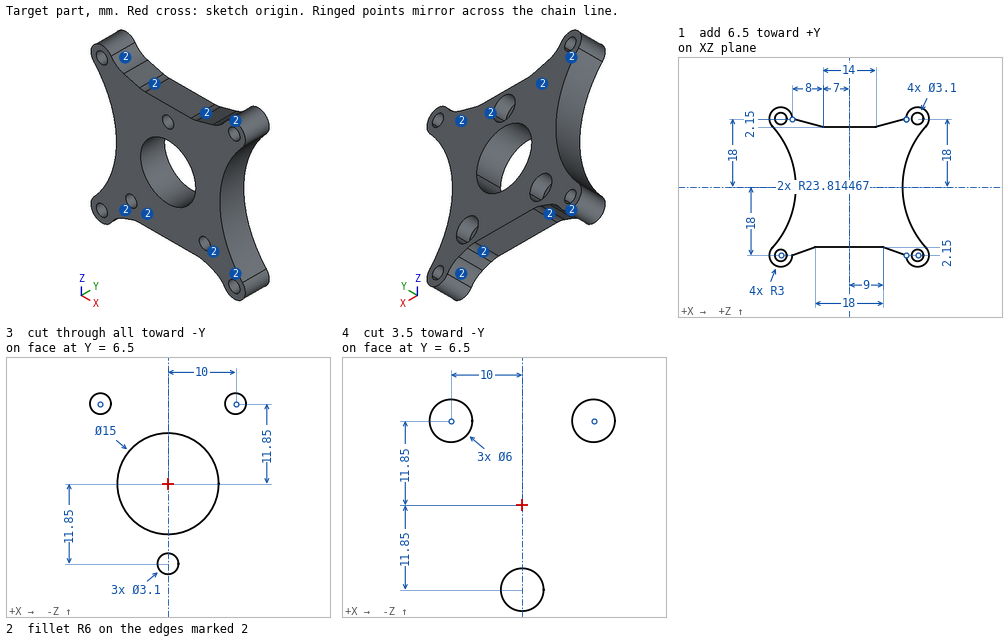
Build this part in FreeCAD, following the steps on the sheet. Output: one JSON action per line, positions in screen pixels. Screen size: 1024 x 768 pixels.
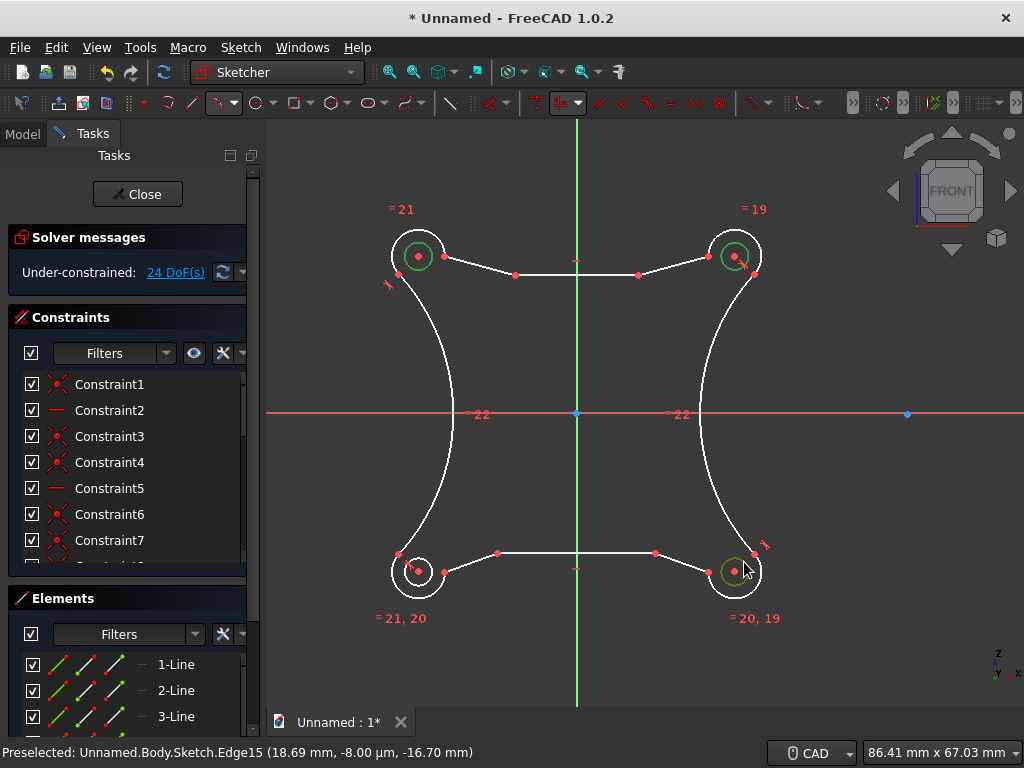
{"action": "left_click", "coordinate": [428, 562]}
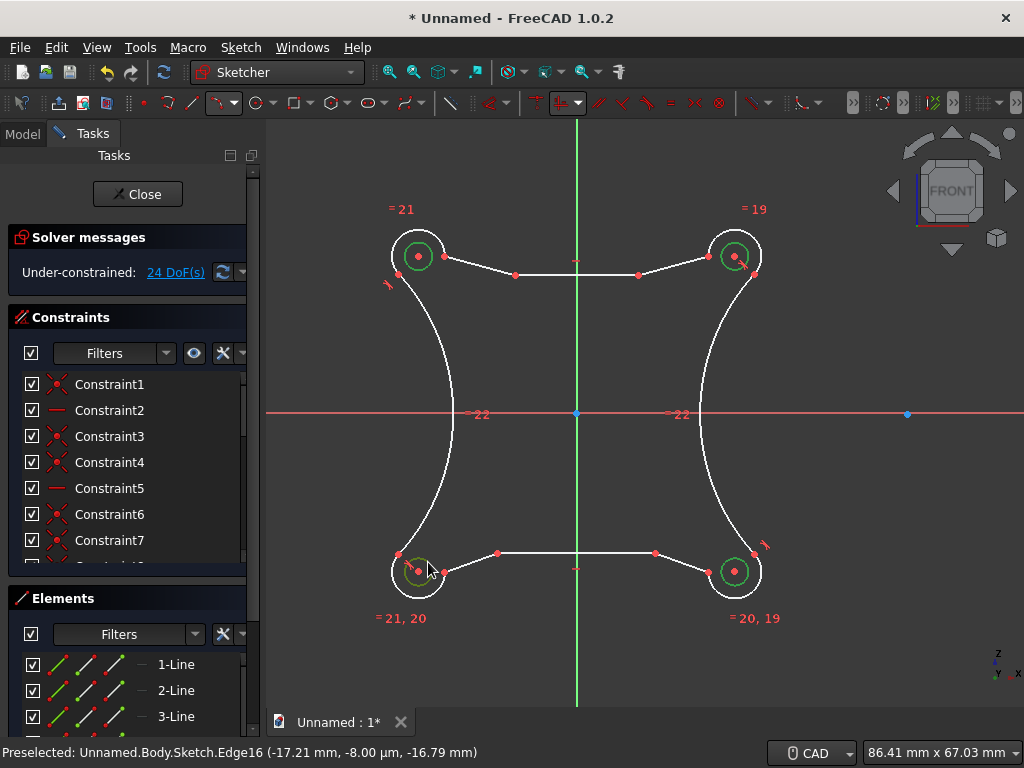
{"action": "left_click", "coordinate": [672, 104]}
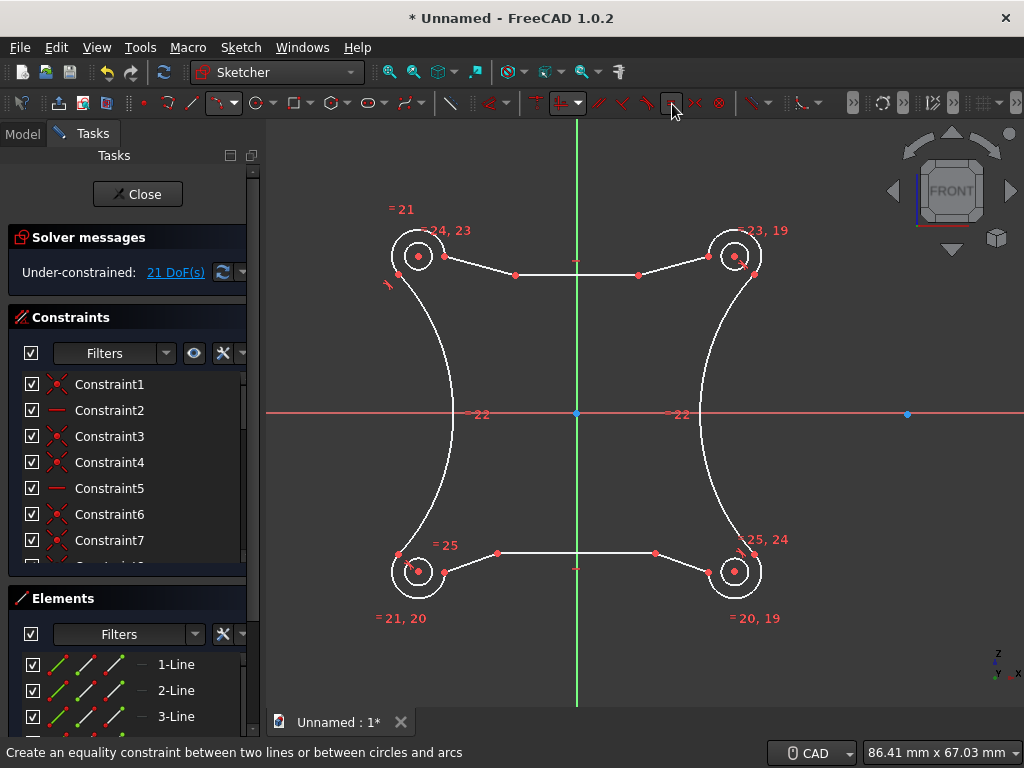
{"action": "scroll", "coordinate": [294, 412], "scroll_direction": "down", "scroll_amount": 1}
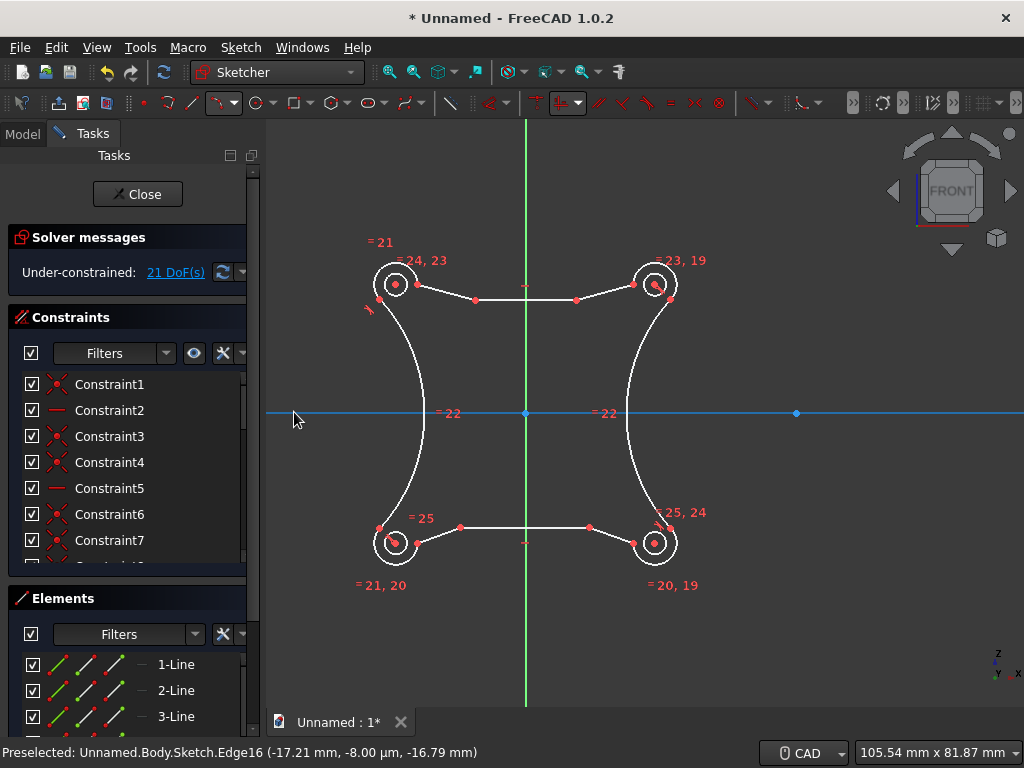
{"action": "left_click", "coordinate": [796, 414]}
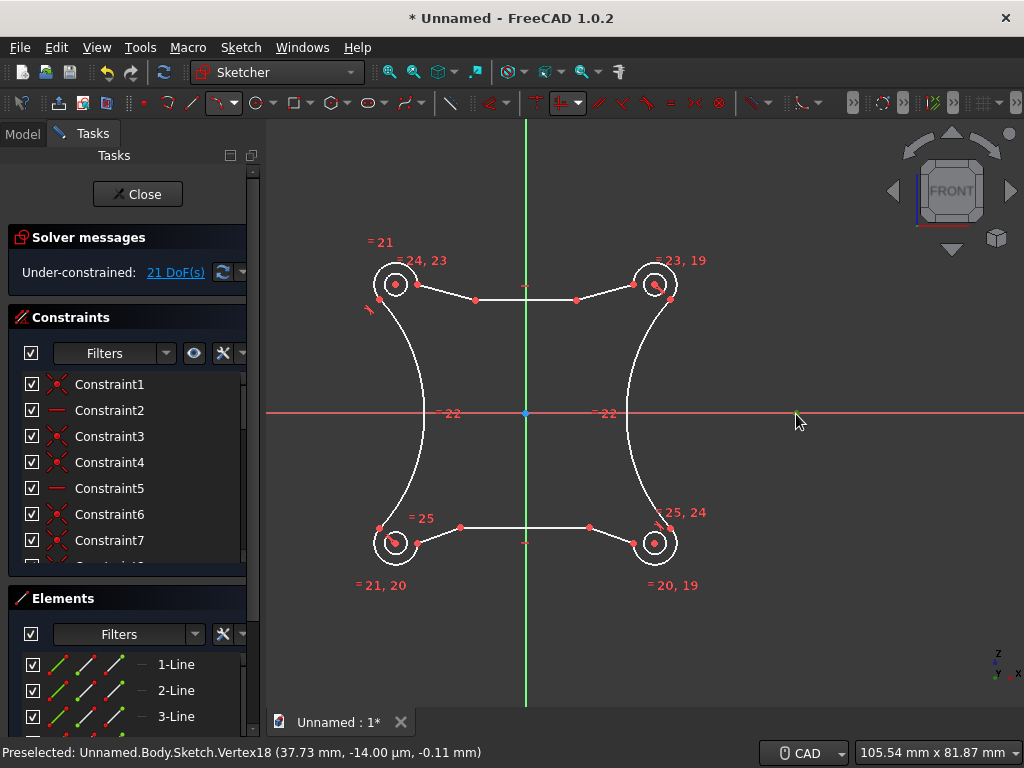
{"action": "left_click", "coordinate": [334, 413]}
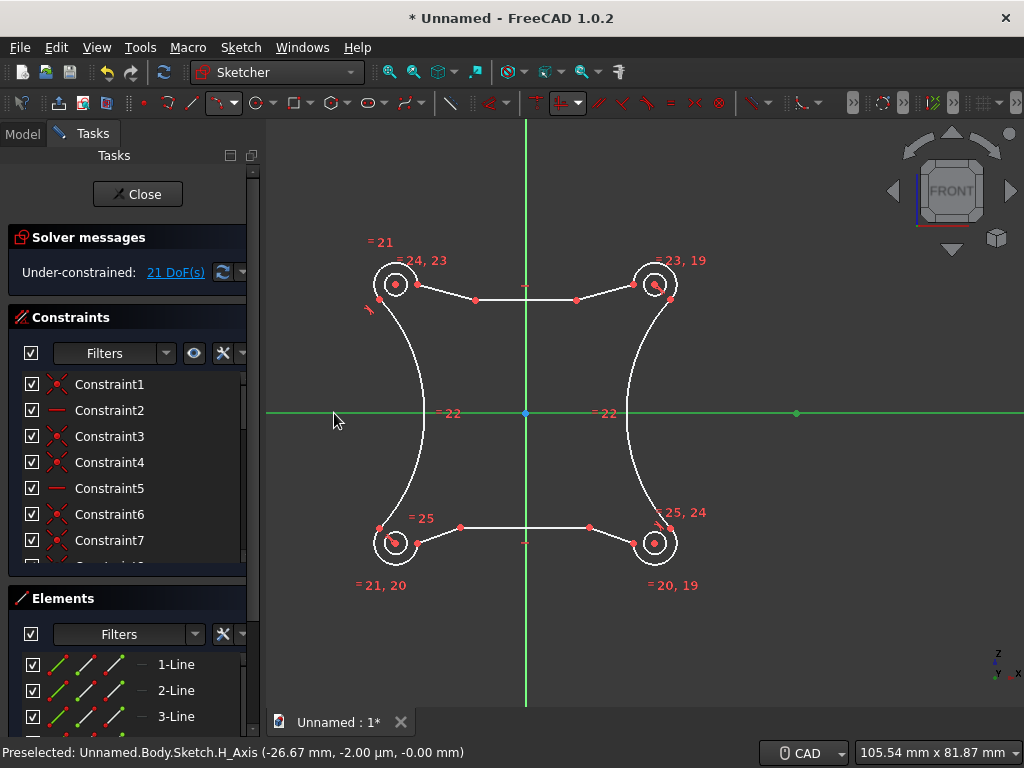
{"action": "left_click", "coordinate": [536, 104]}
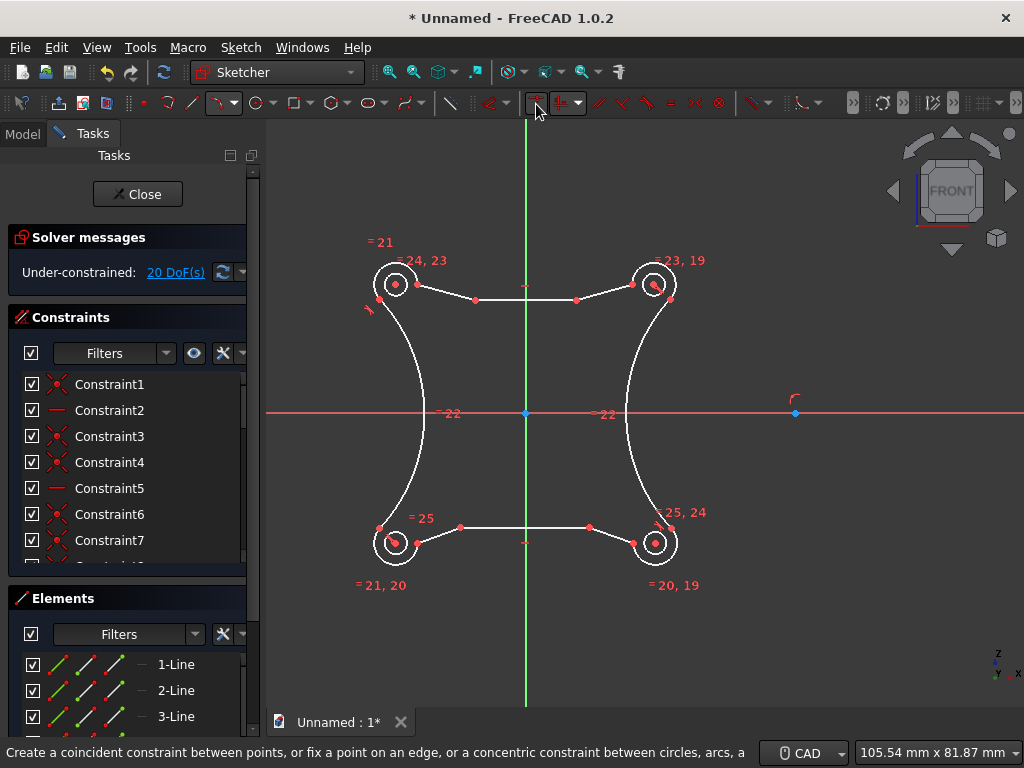
{"action": "scroll", "coordinate": [859, 413], "scroll_direction": "down", "scroll_amount": 1}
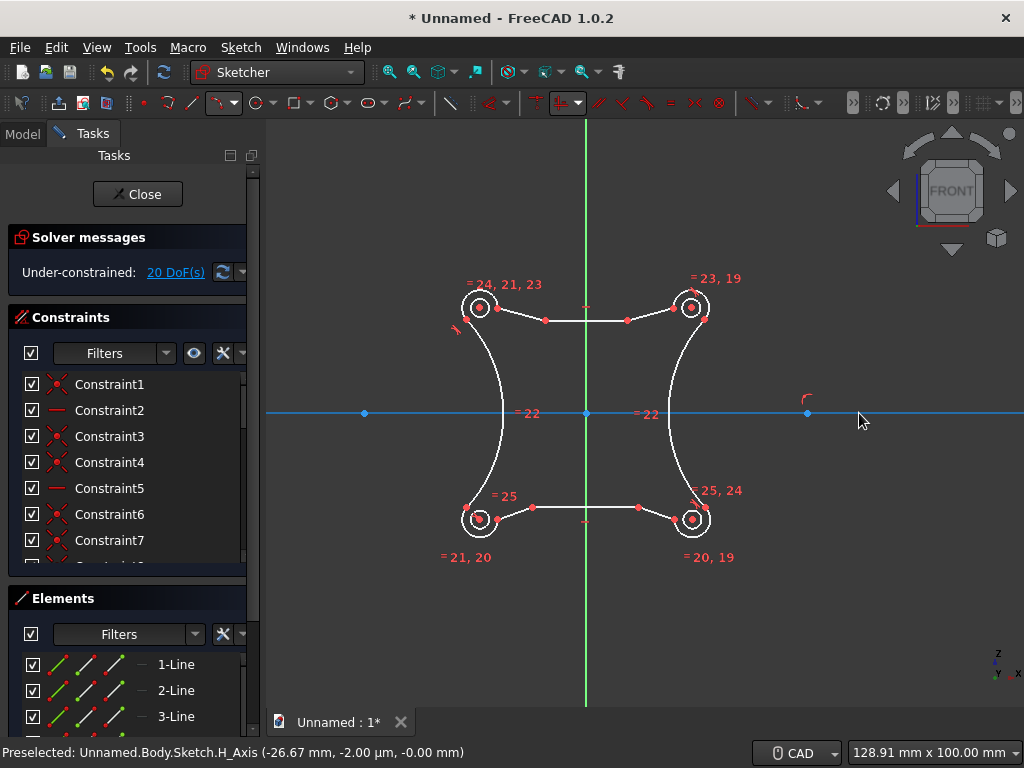
{"action": "left_click", "coordinate": [364, 414]}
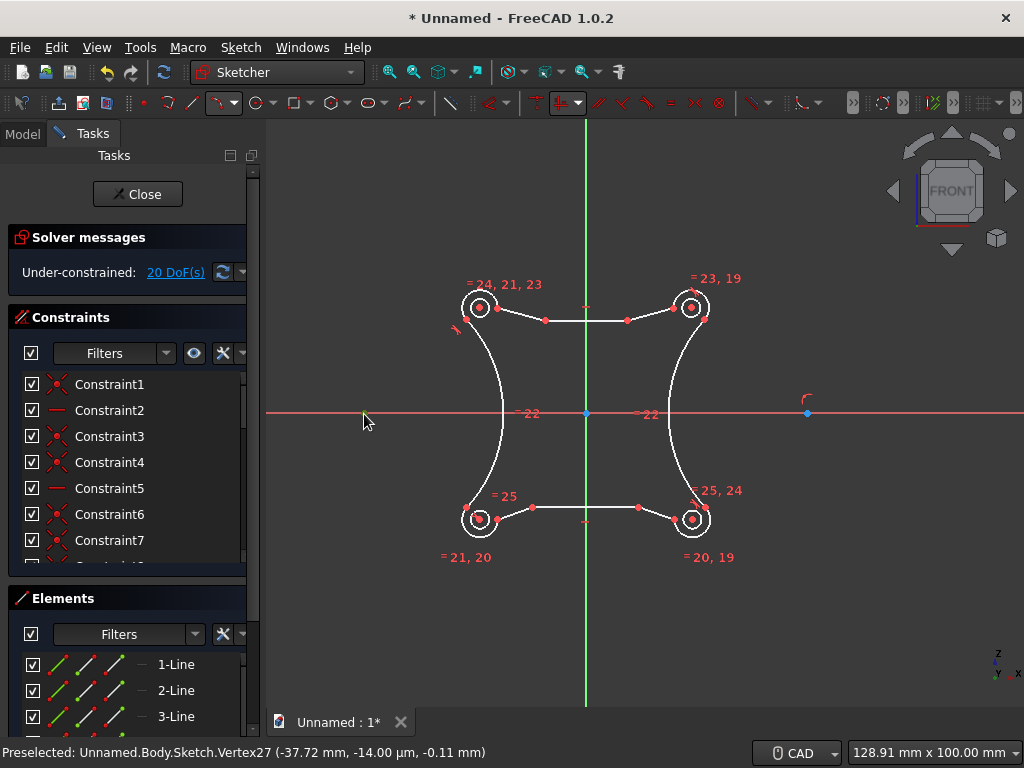
{"action": "left_click", "coordinate": [334, 413]}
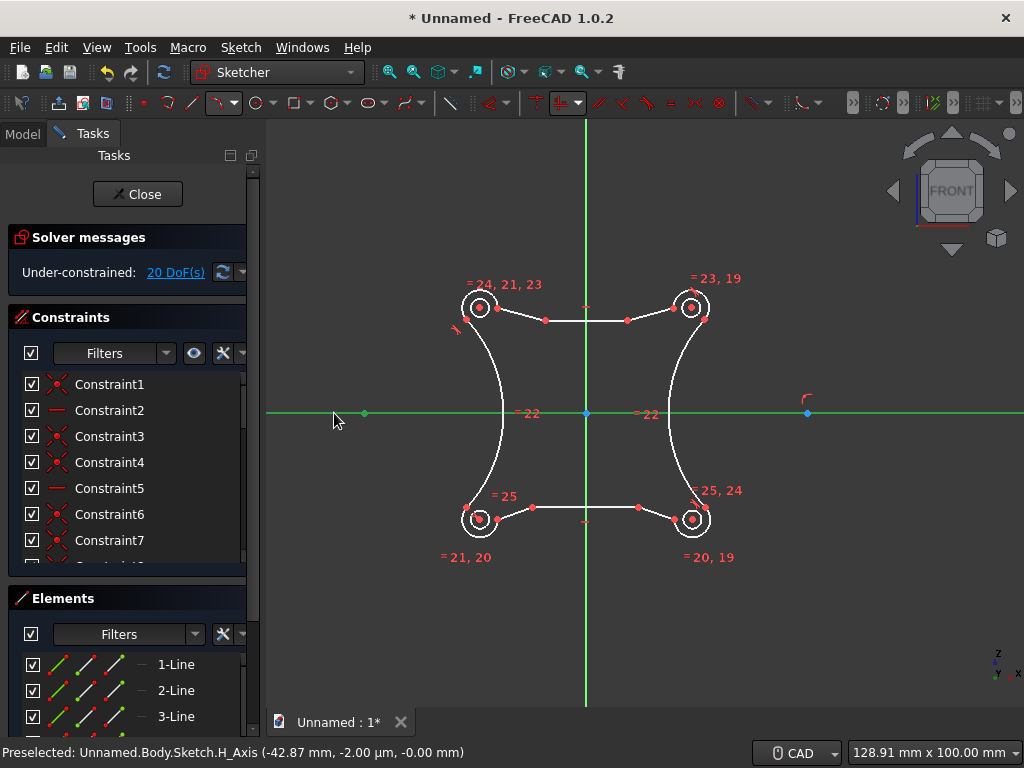
{"action": "left_click", "coordinate": [536, 104]}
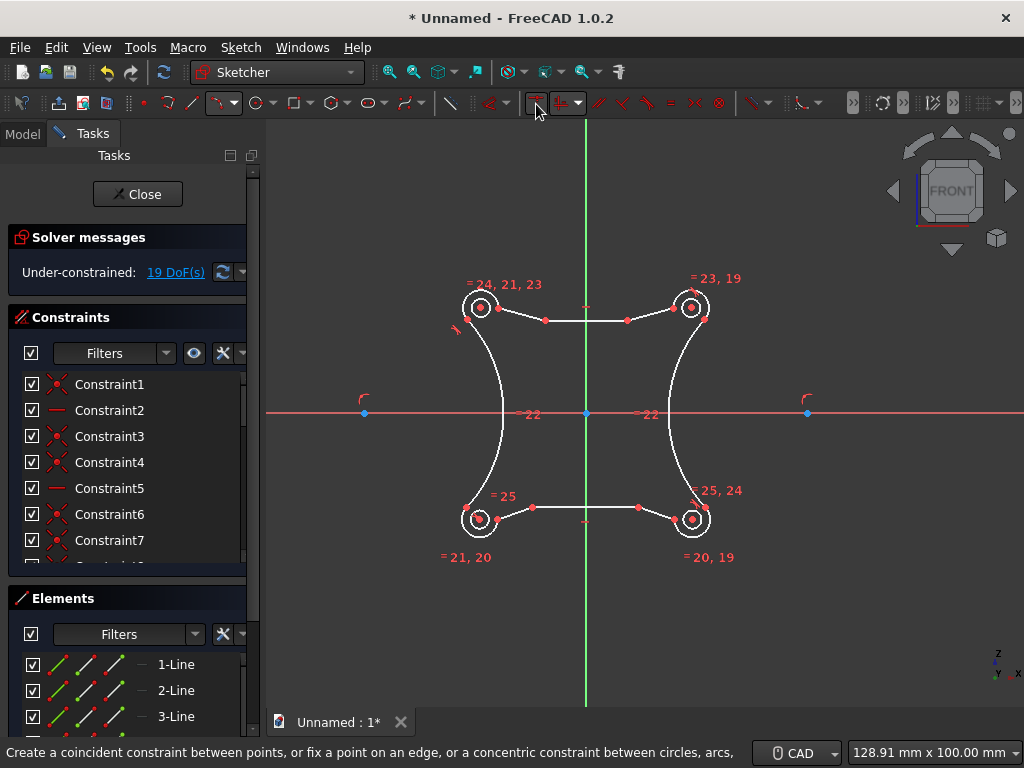
{"action": "left_click", "coordinate": [692, 520]}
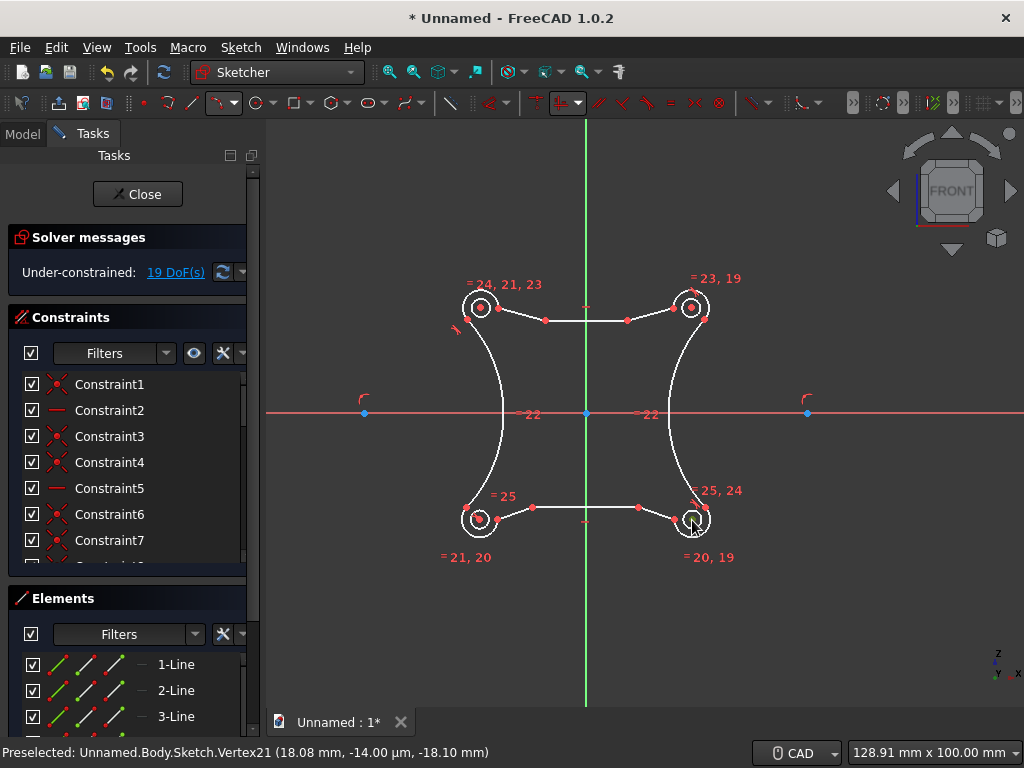
{"action": "left_click", "coordinate": [480, 520]}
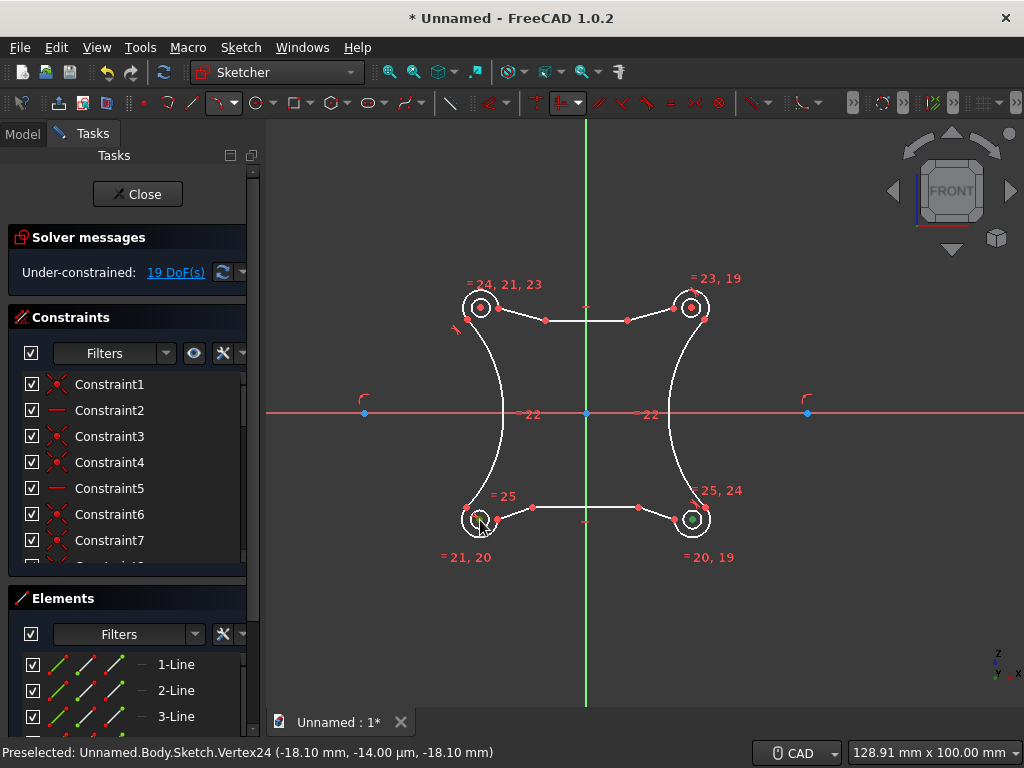
{"action": "left_click", "coordinate": [586, 641]}